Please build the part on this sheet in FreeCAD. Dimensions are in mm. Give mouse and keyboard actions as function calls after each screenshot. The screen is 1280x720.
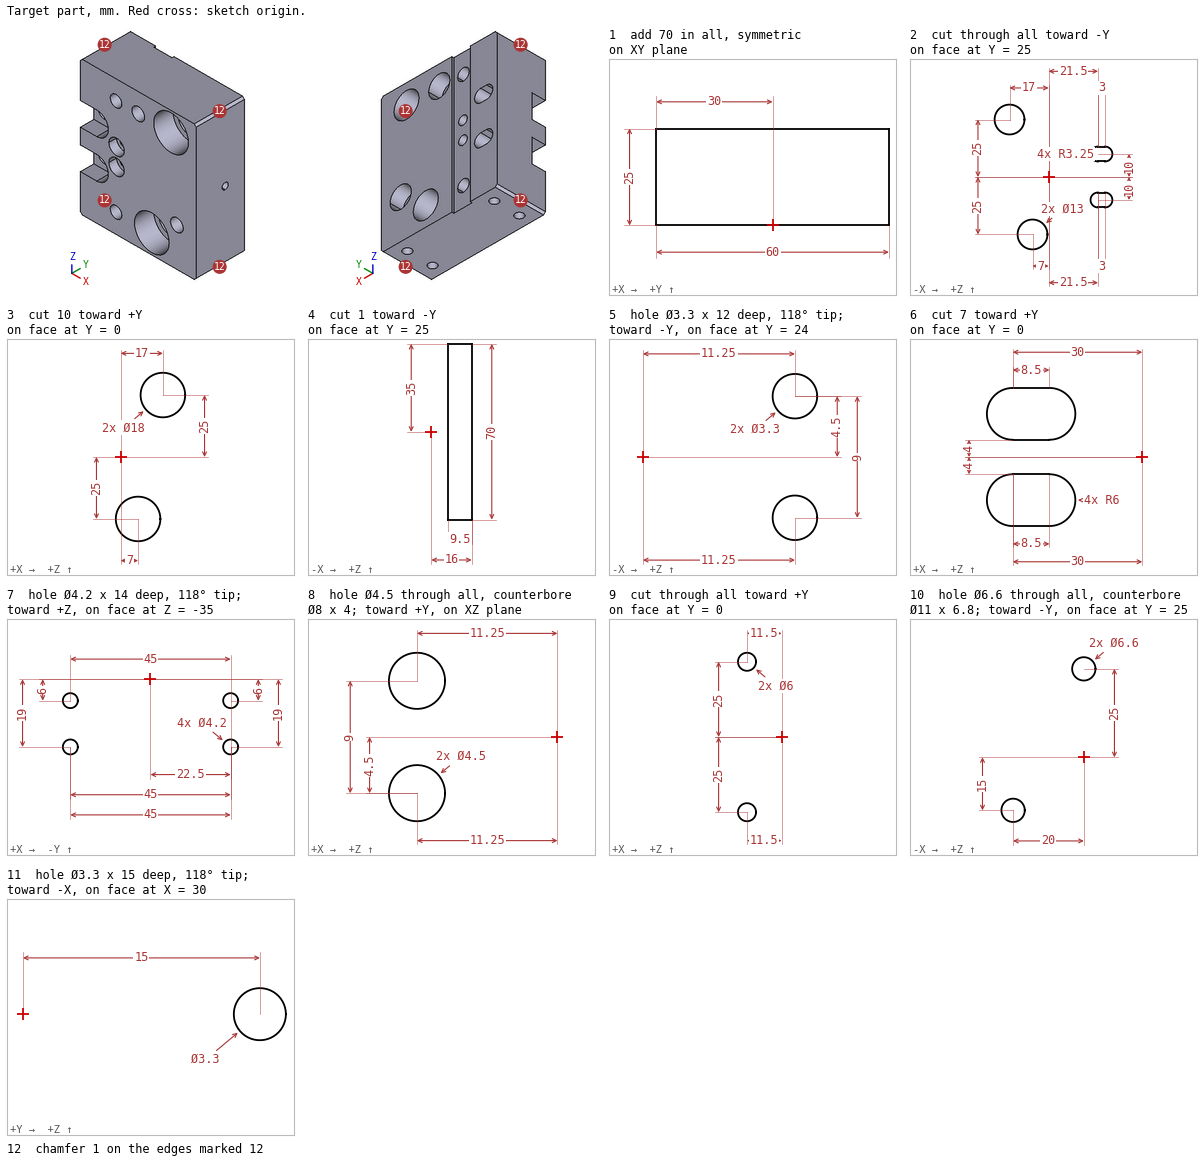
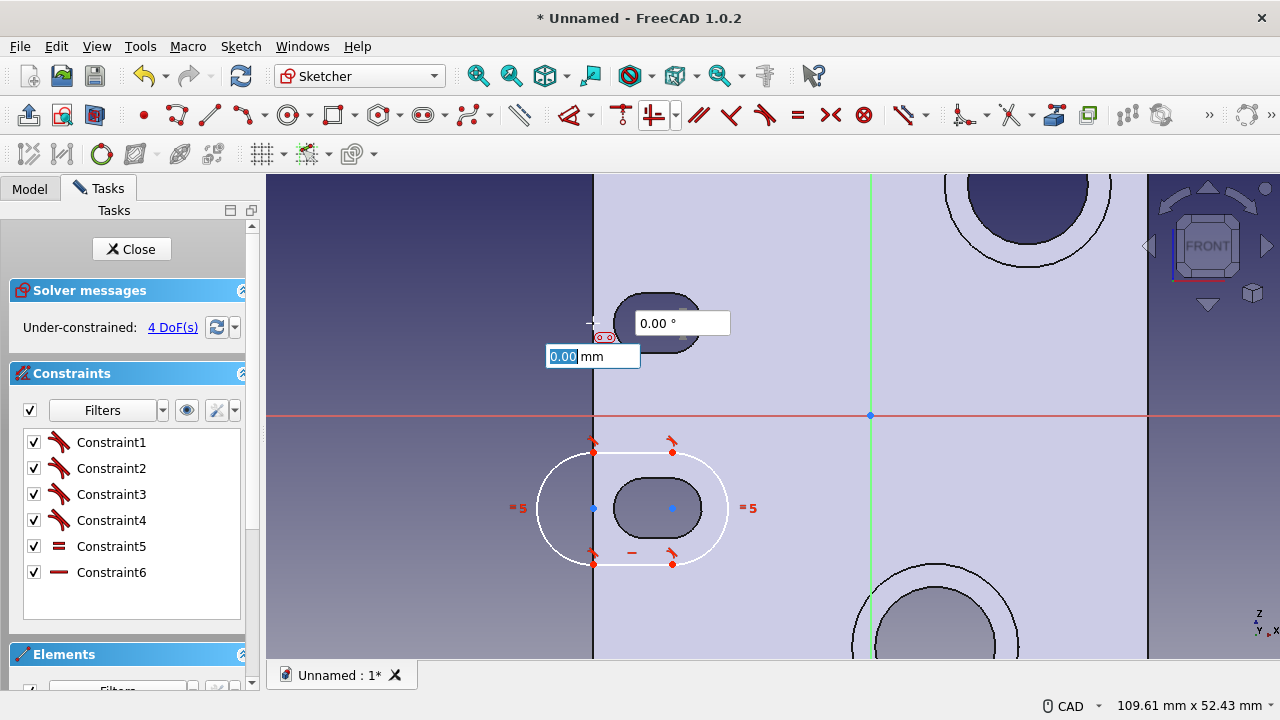
click(672, 323)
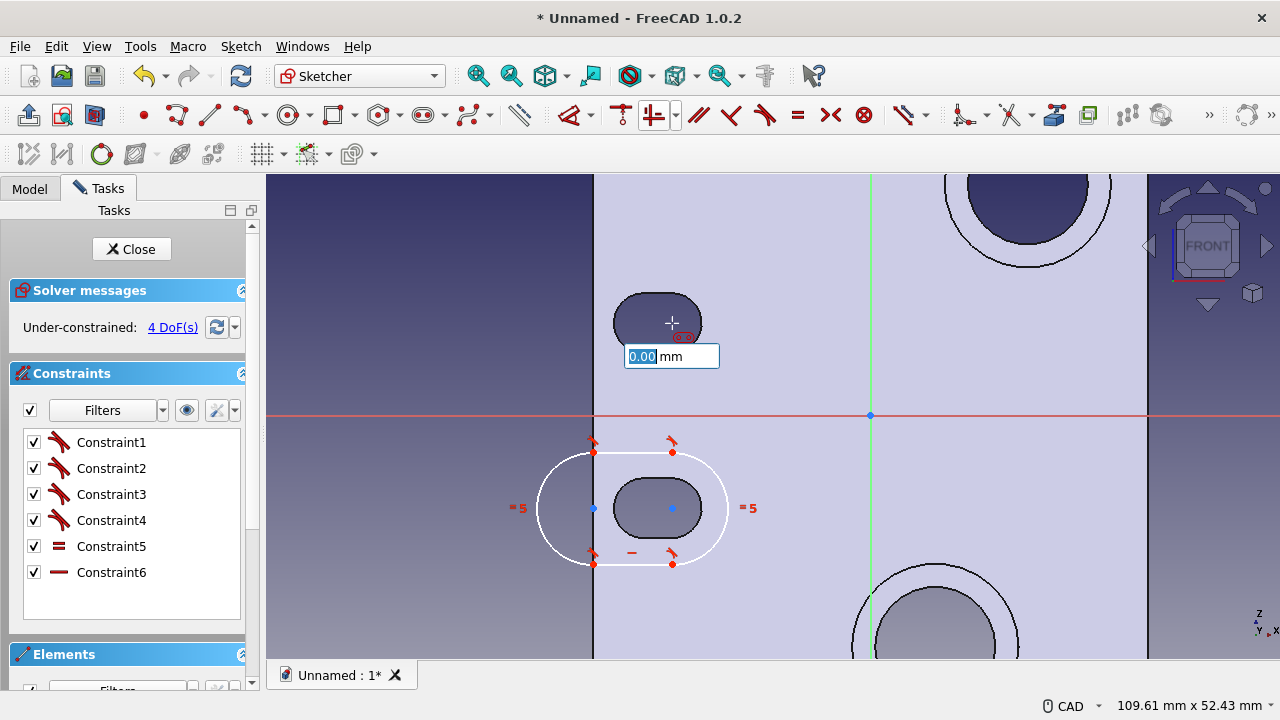
click(632, 379)
key(Escape)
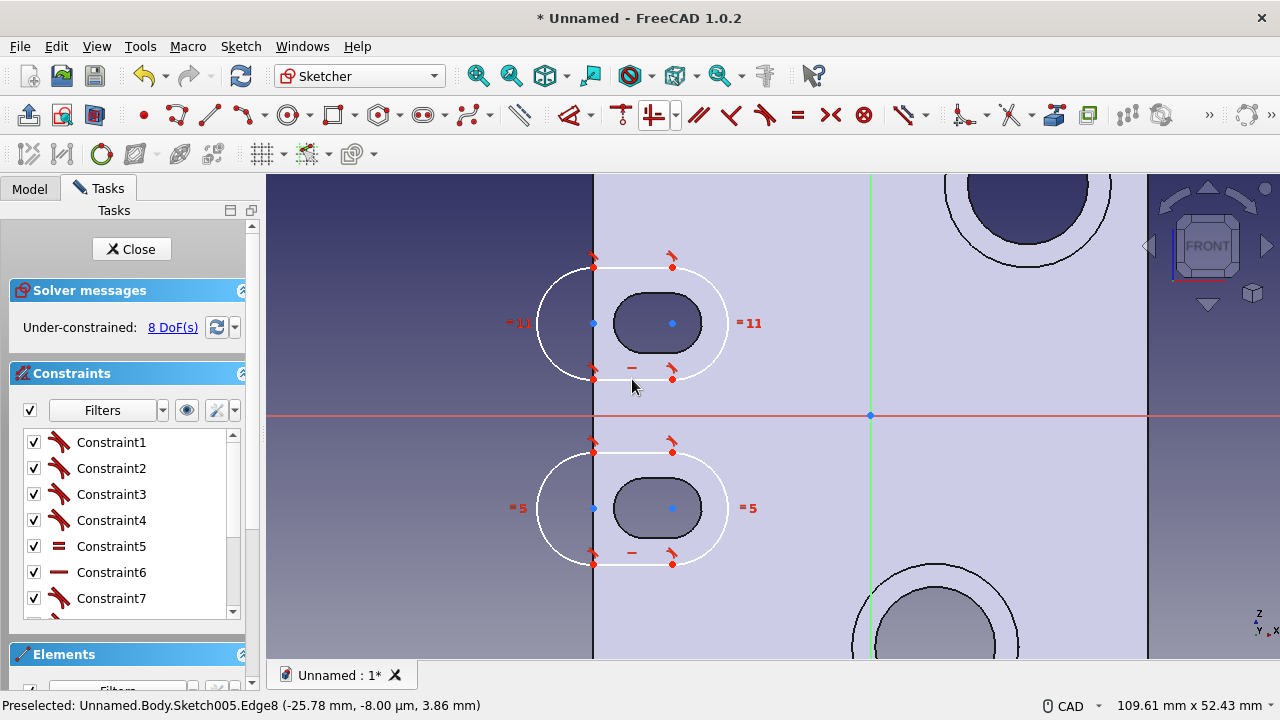
click(548, 476)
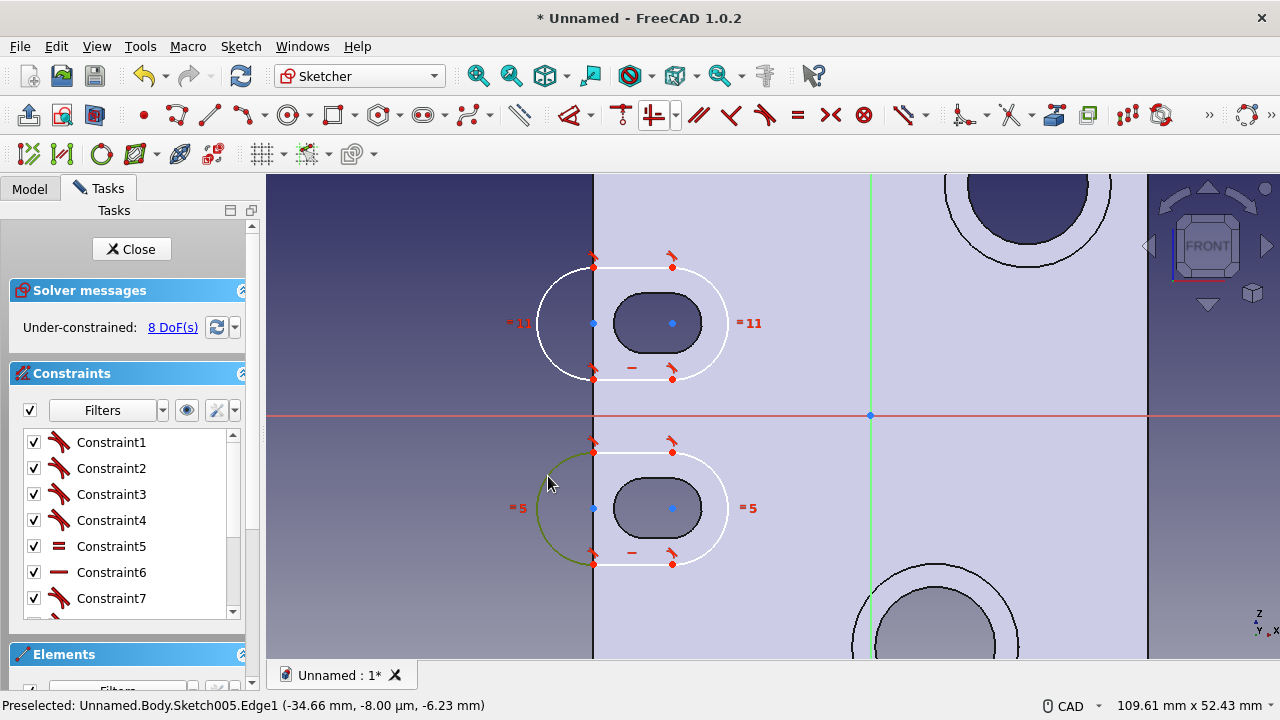
click(548, 291)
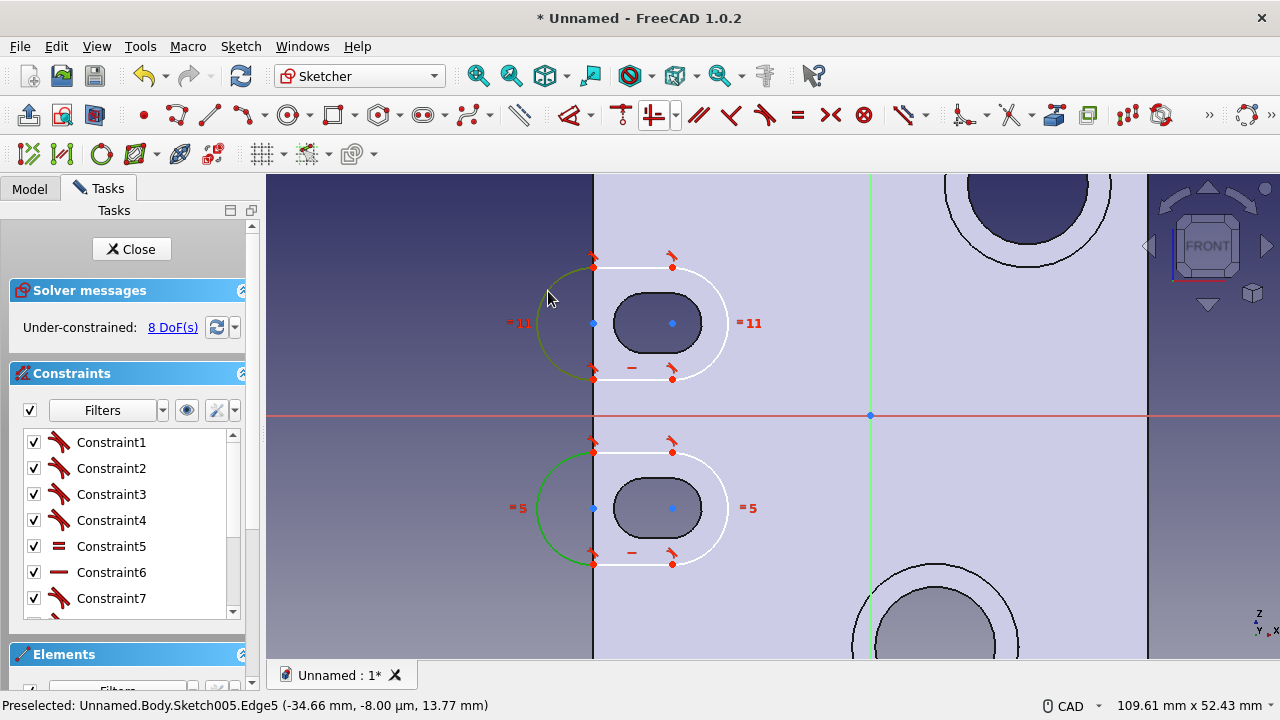
click(798, 116)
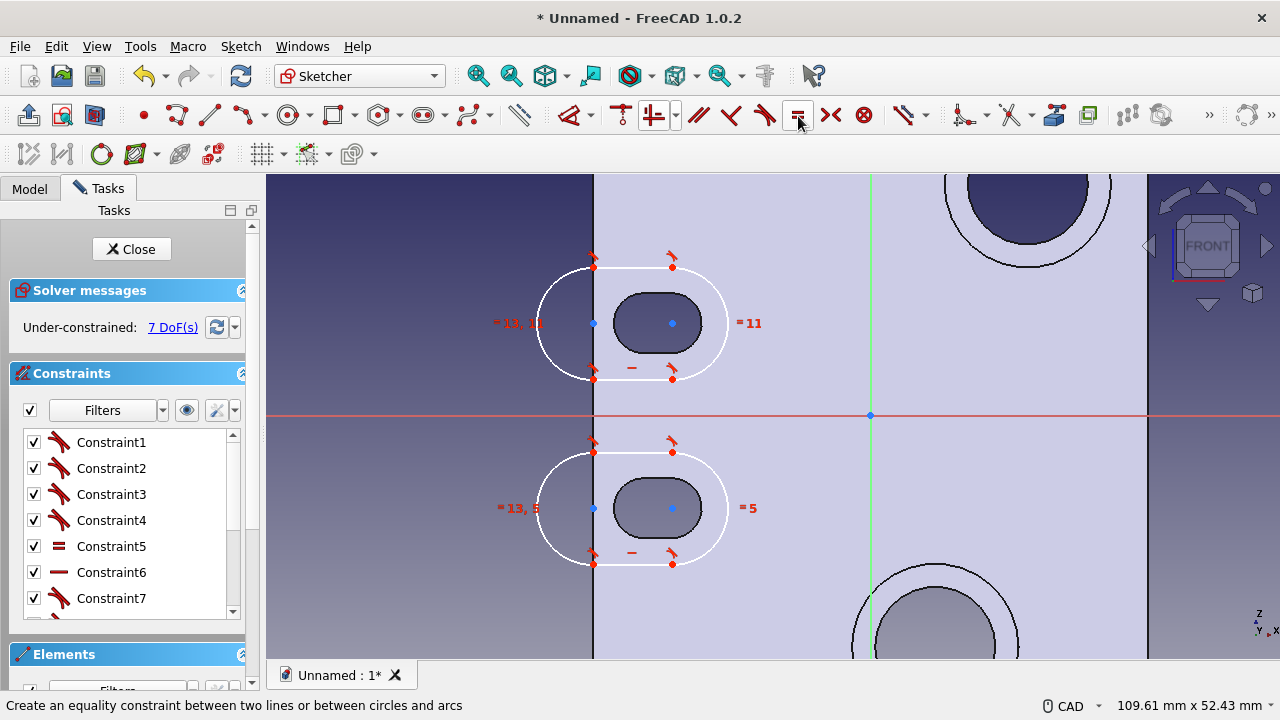
key(d)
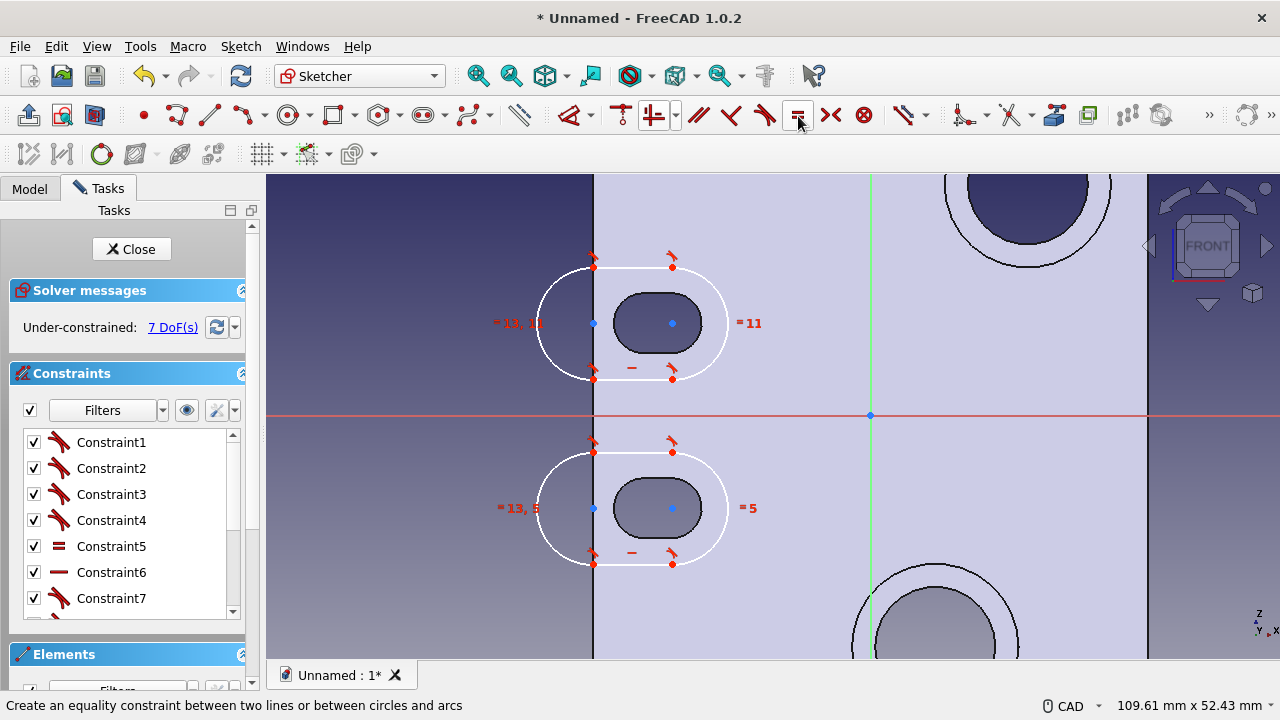
click(548, 476)
click(522, 457)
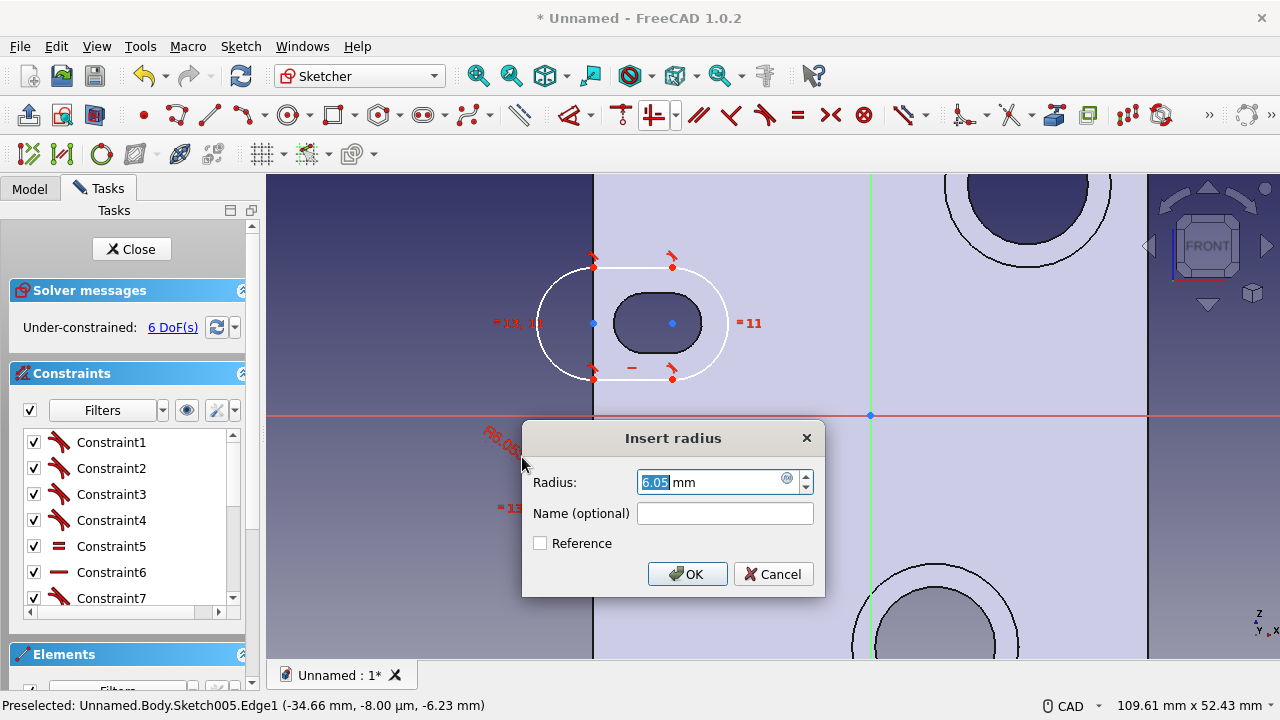
text(6)
key(Return)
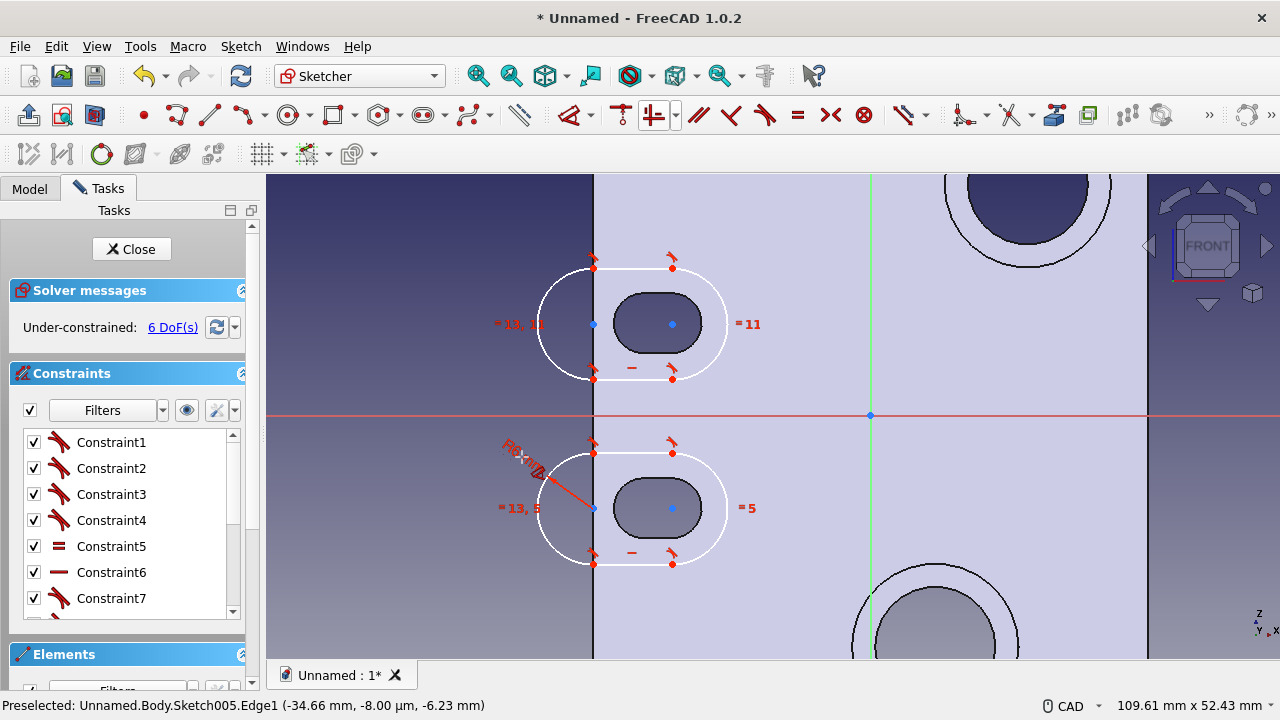
click(593, 453)
click(905, 435)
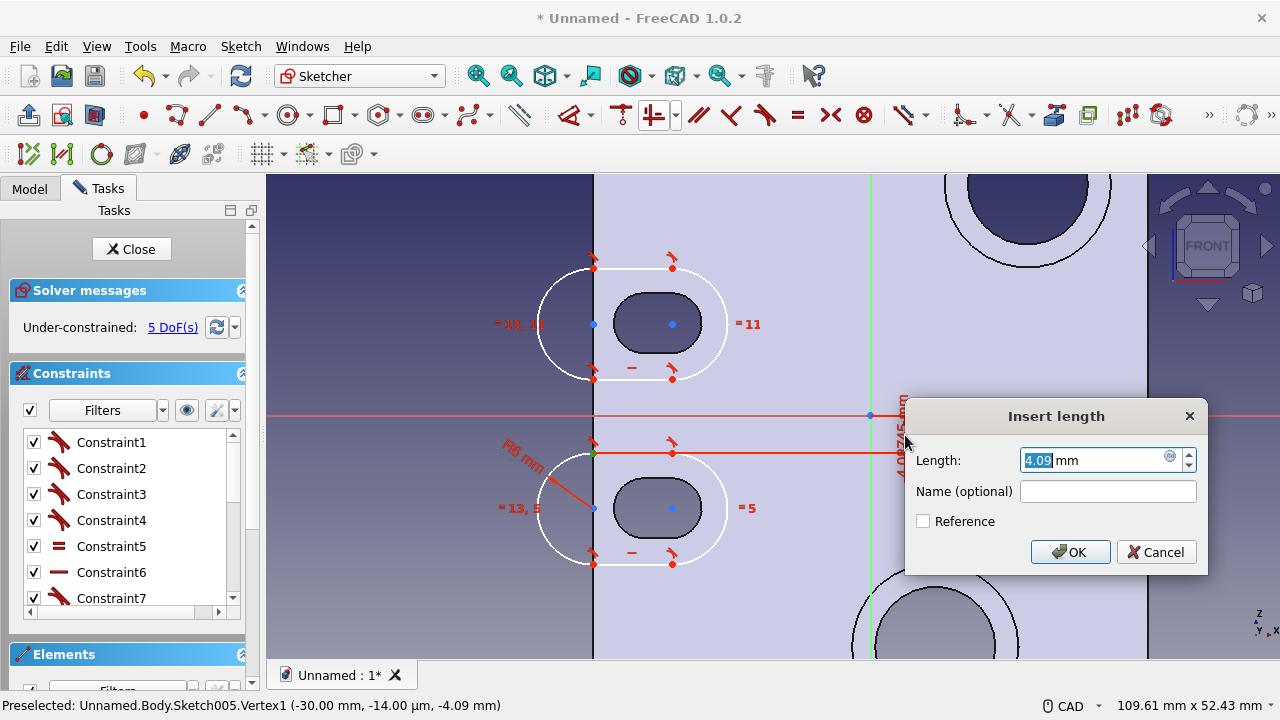
text(4)
key(Return)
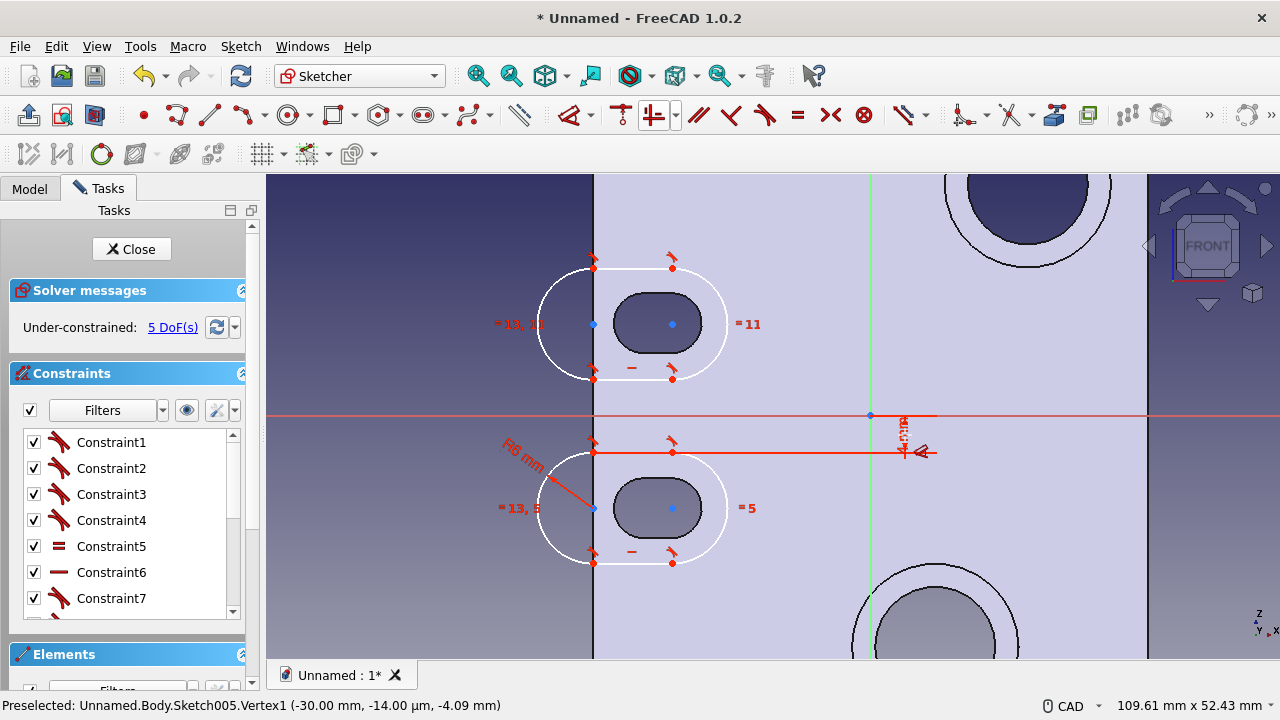
click(593, 380)
click(905, 398)